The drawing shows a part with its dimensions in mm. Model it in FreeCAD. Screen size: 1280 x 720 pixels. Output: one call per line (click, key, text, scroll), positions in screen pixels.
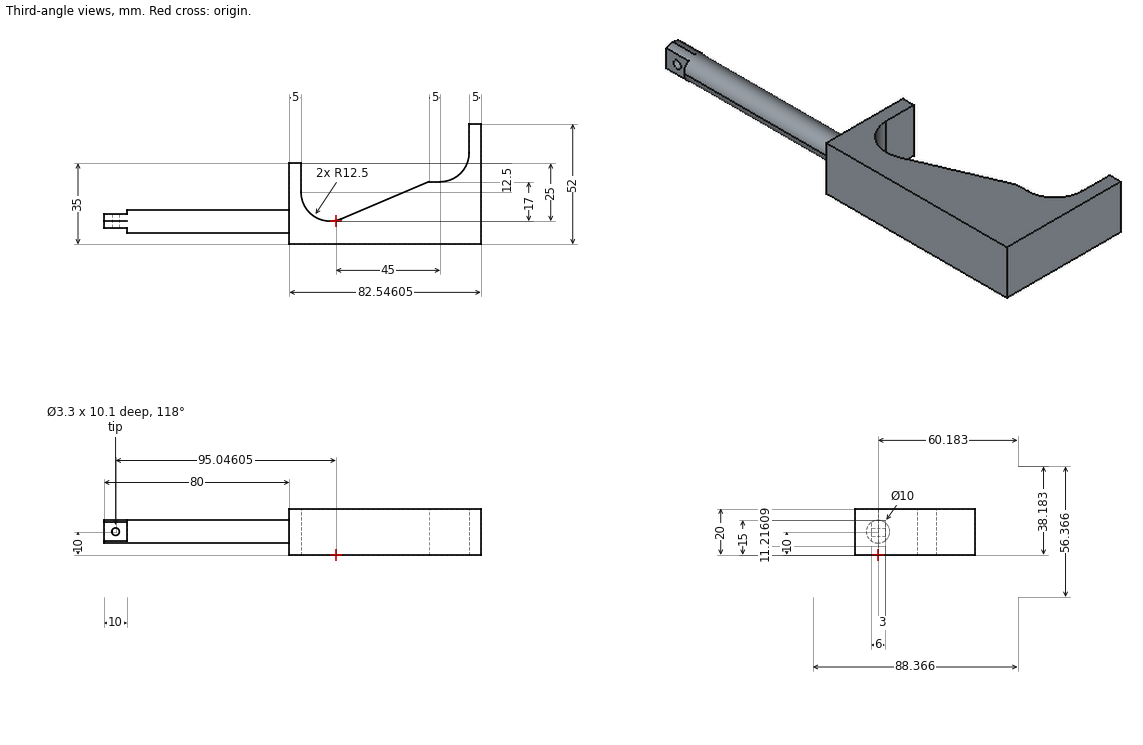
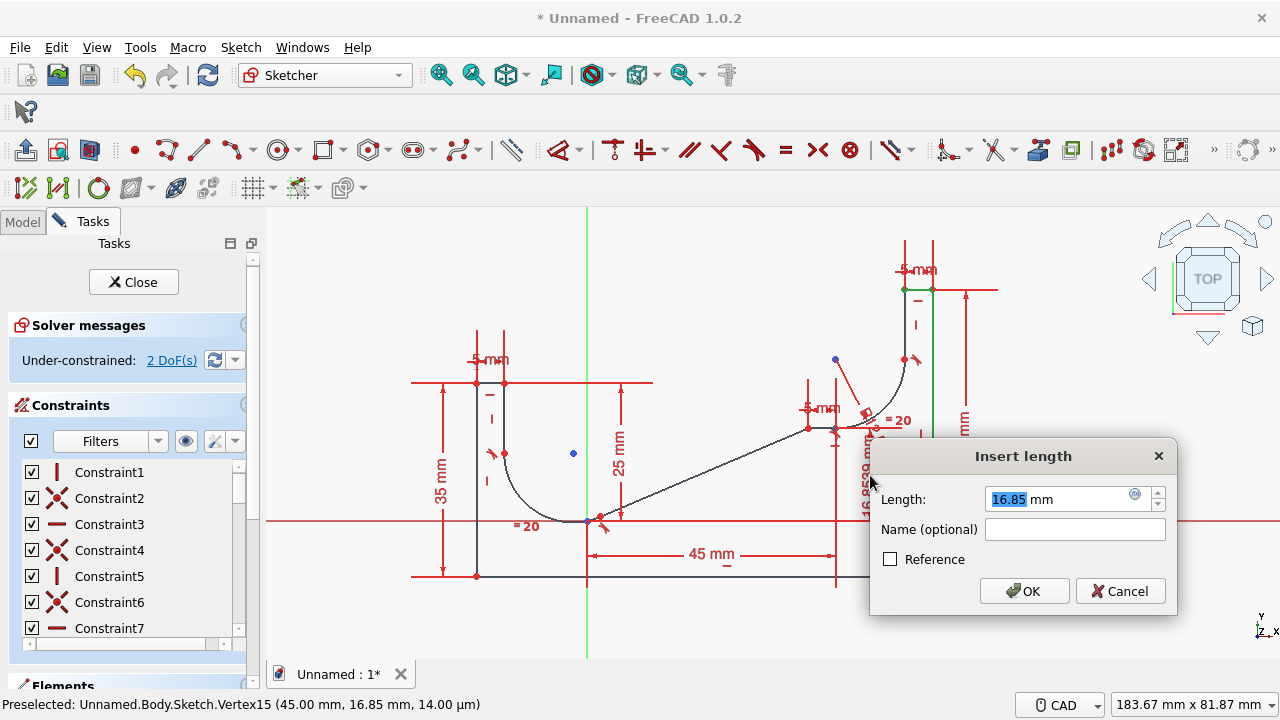
text(17)
key(Return)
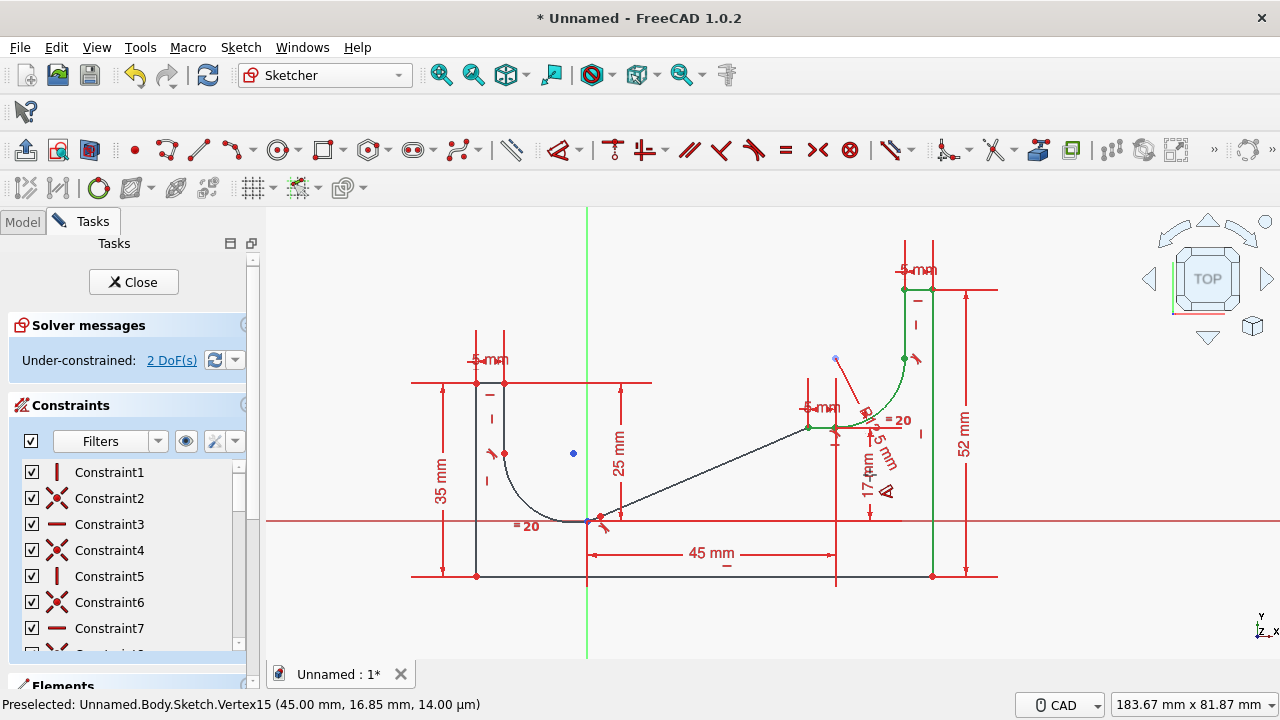
click(504, 432)
click(538, 418)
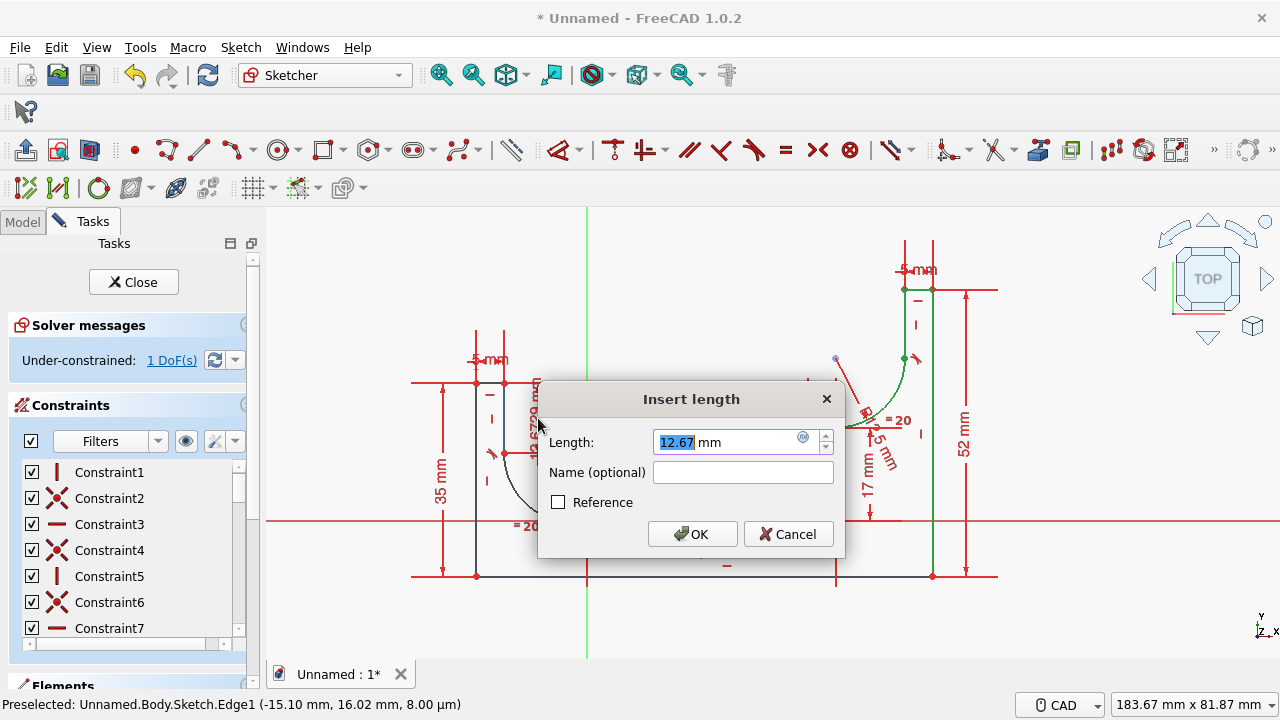
text(12.5)
key(Return)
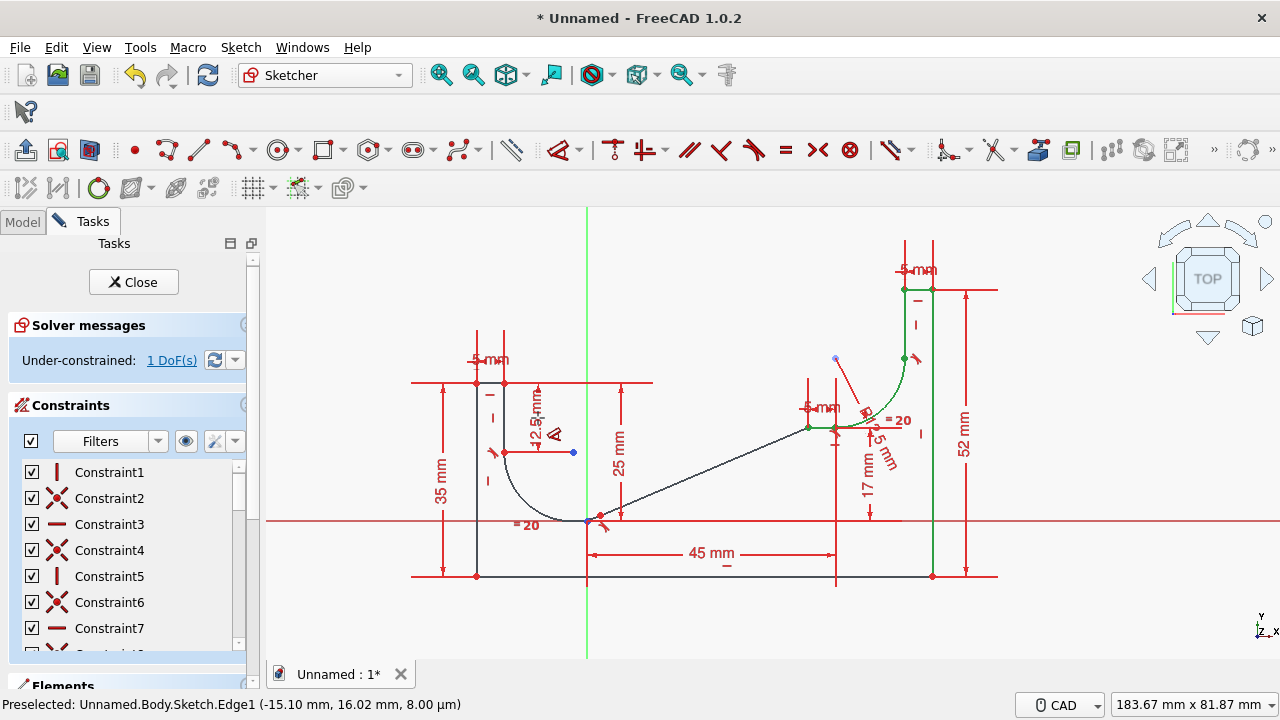
click(613, 577)
click(705, 611)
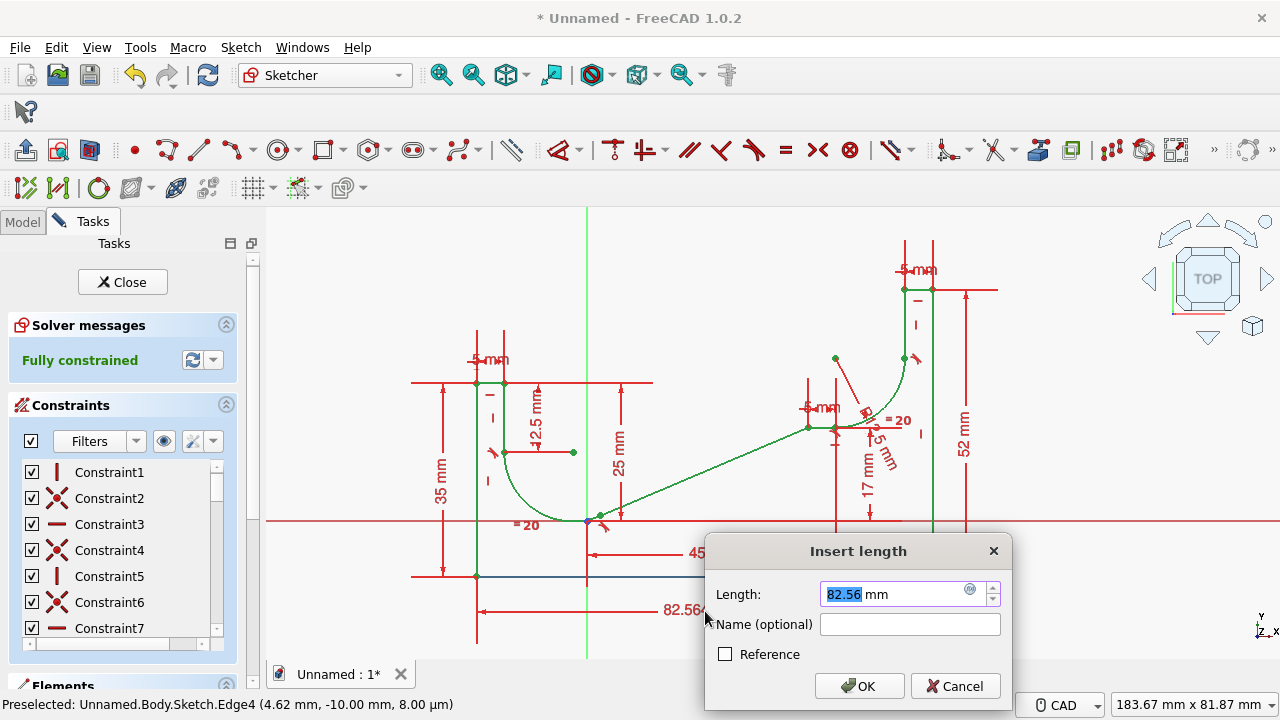
text(82.54605)
key(Return)
key(Escape)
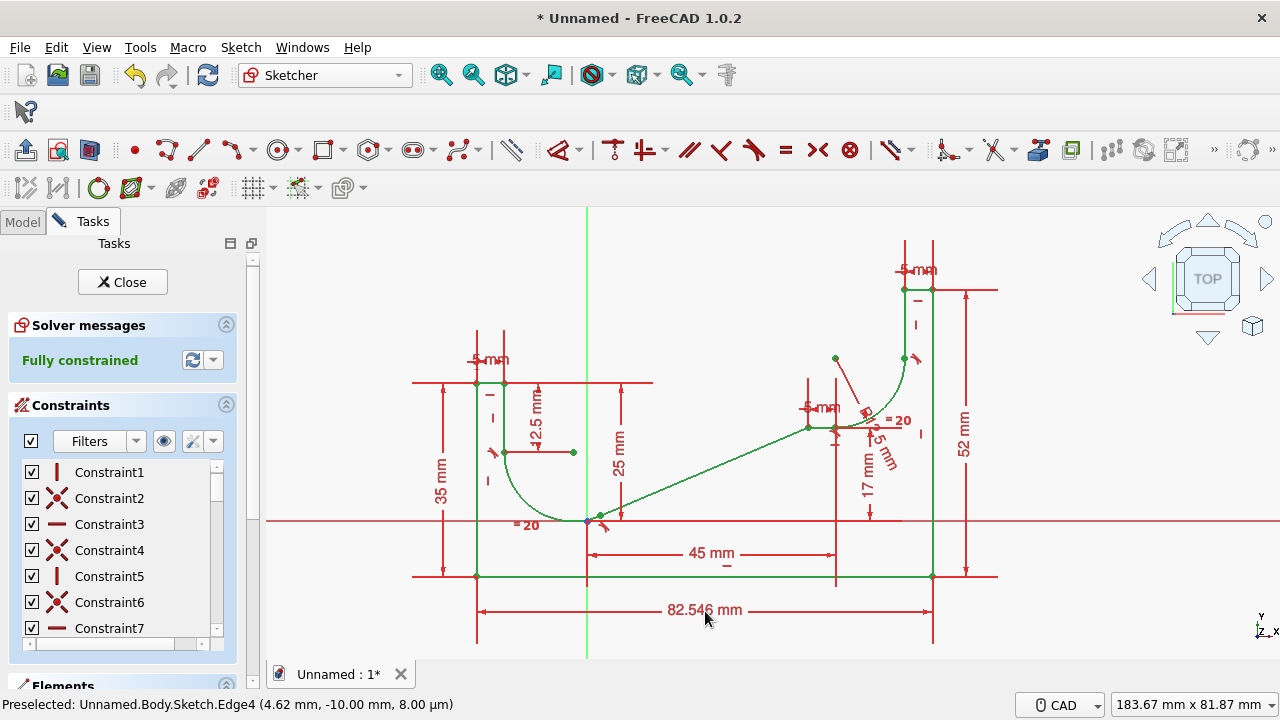
click(123, 282)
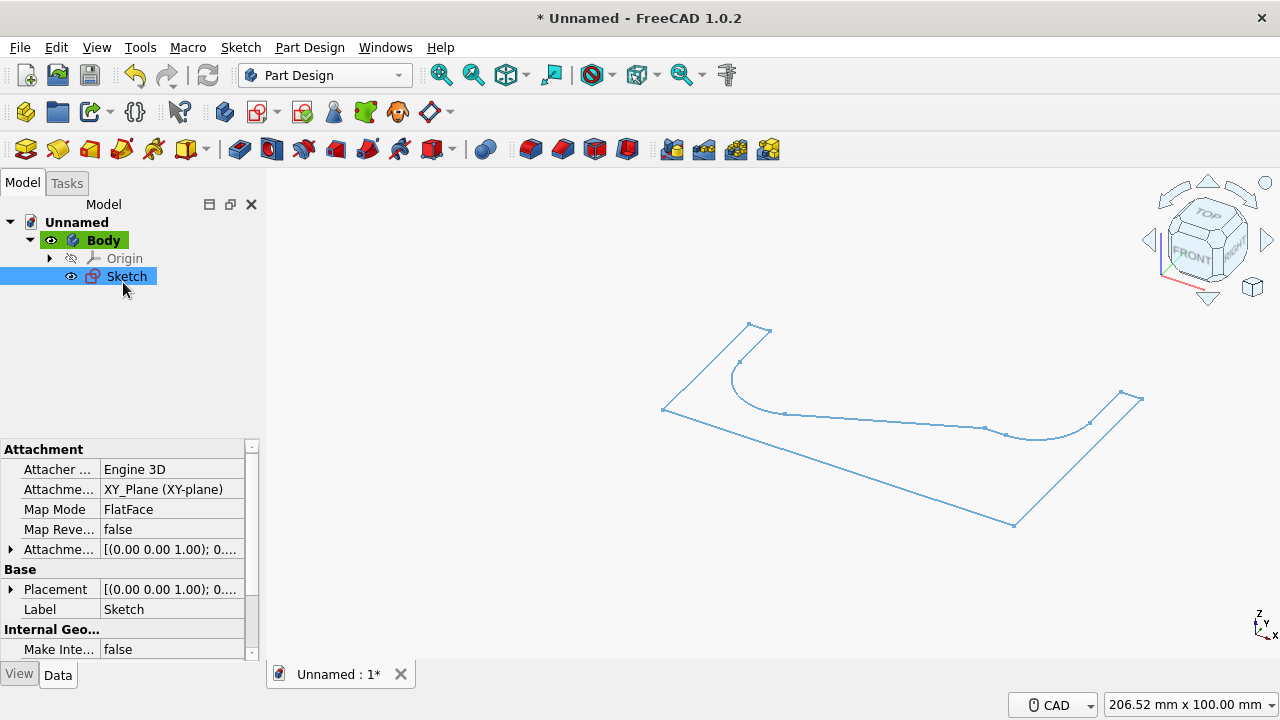
click(26, 150)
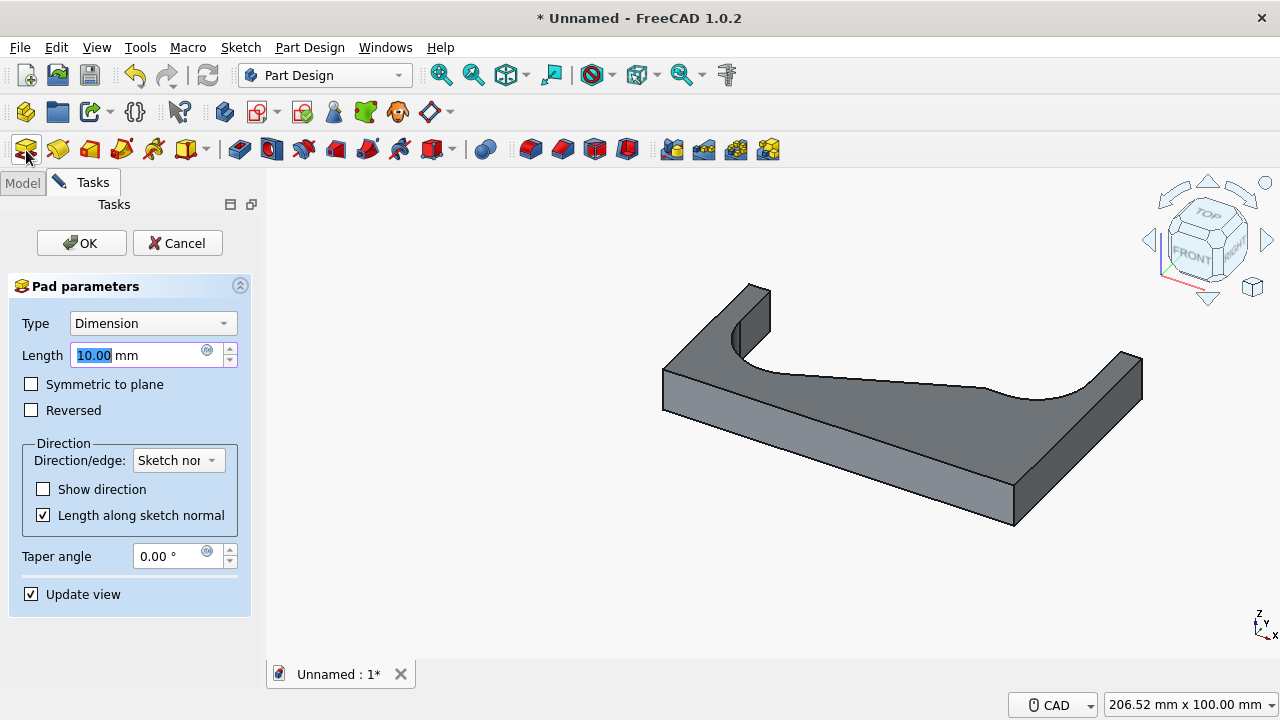
text(20)
key(Tab)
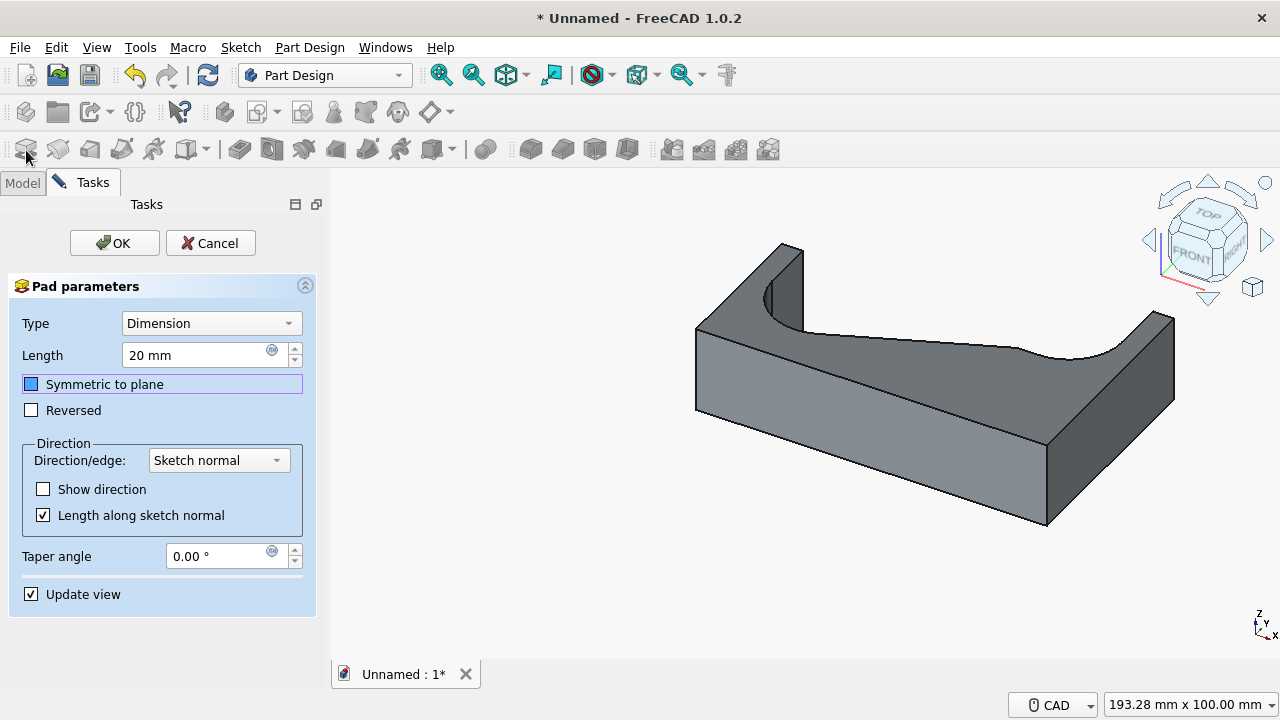
click(115, 243)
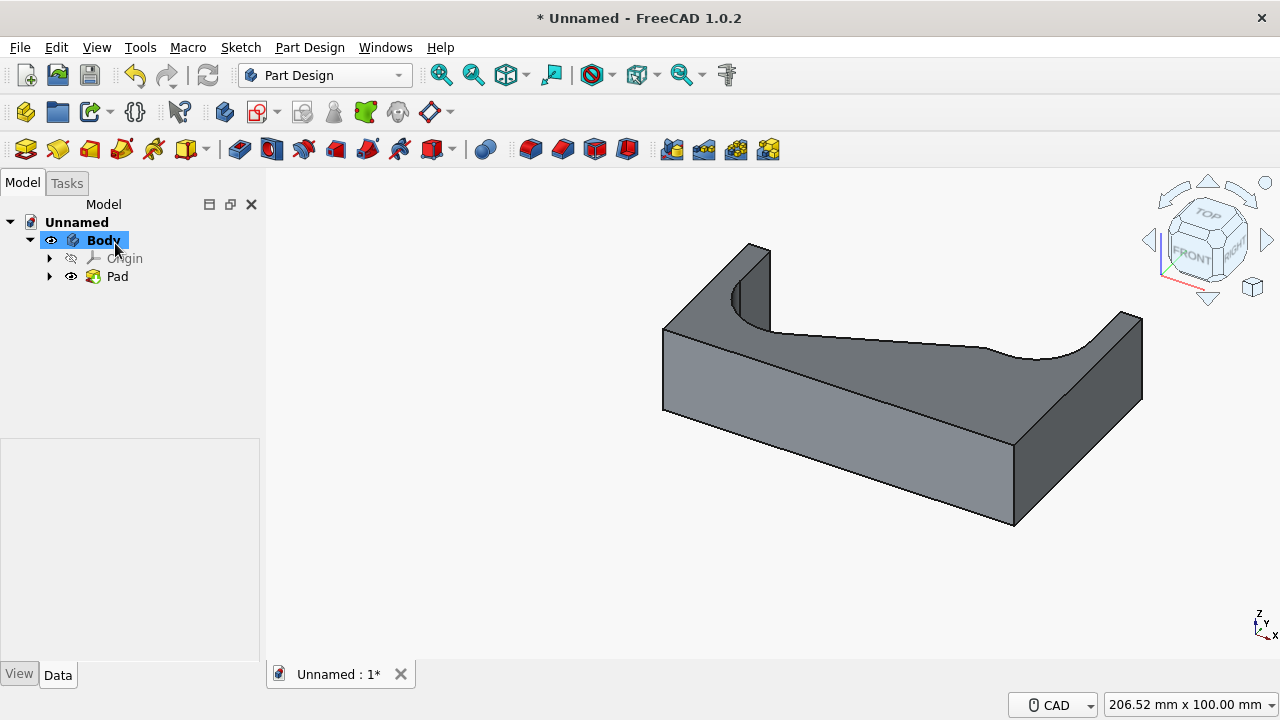
key(6)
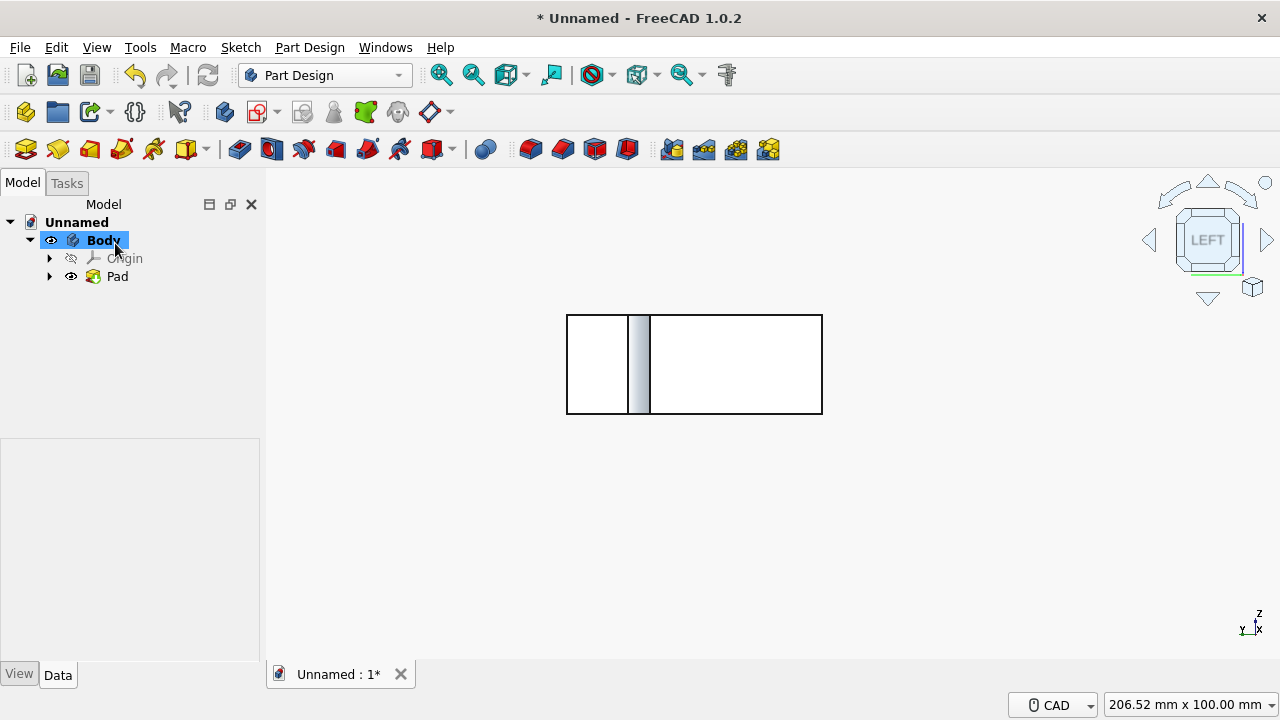
click(442, 76)